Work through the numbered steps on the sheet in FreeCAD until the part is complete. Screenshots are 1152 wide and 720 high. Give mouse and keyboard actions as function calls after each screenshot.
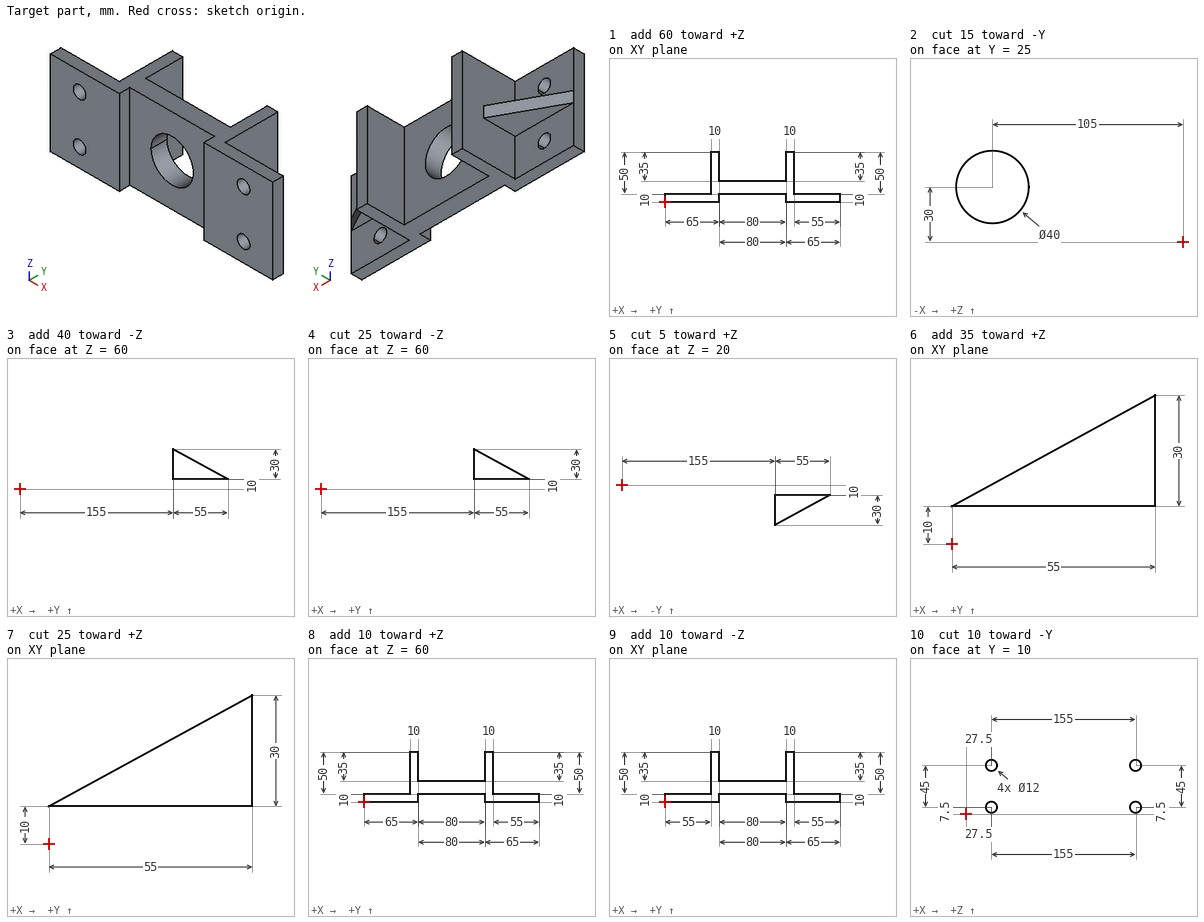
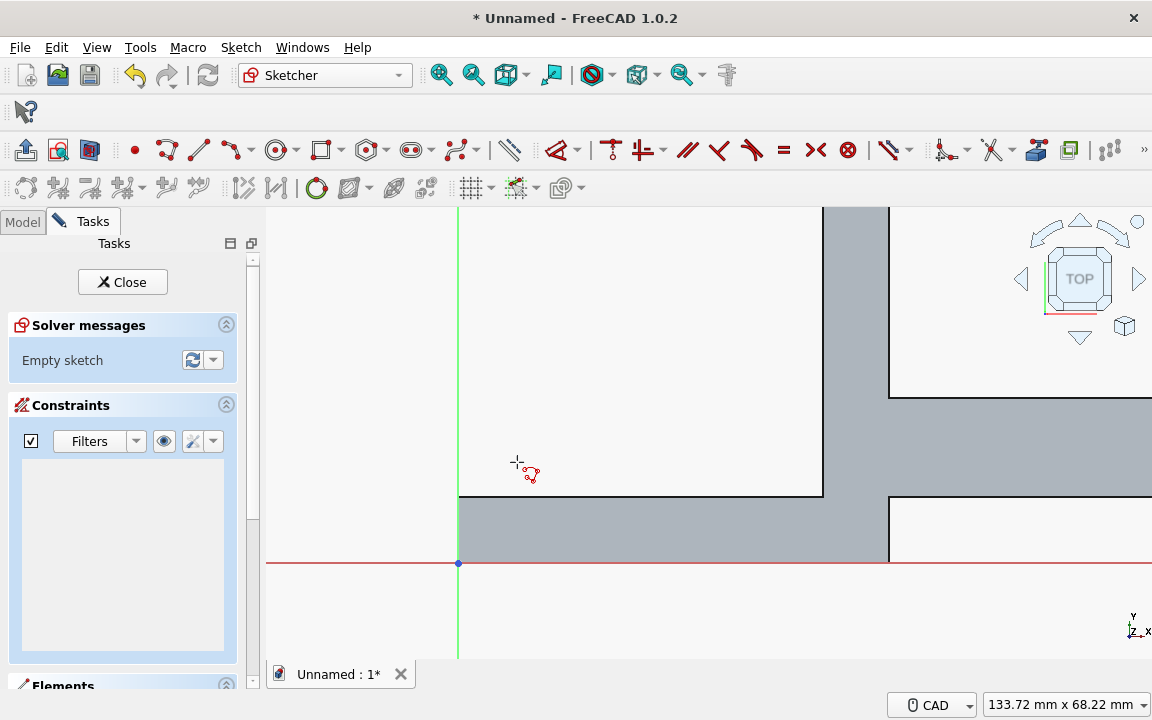
click(458, 497)
click(823, 298)
click(823, 497)
click(458, 498)
key(Escape)
key(Escape)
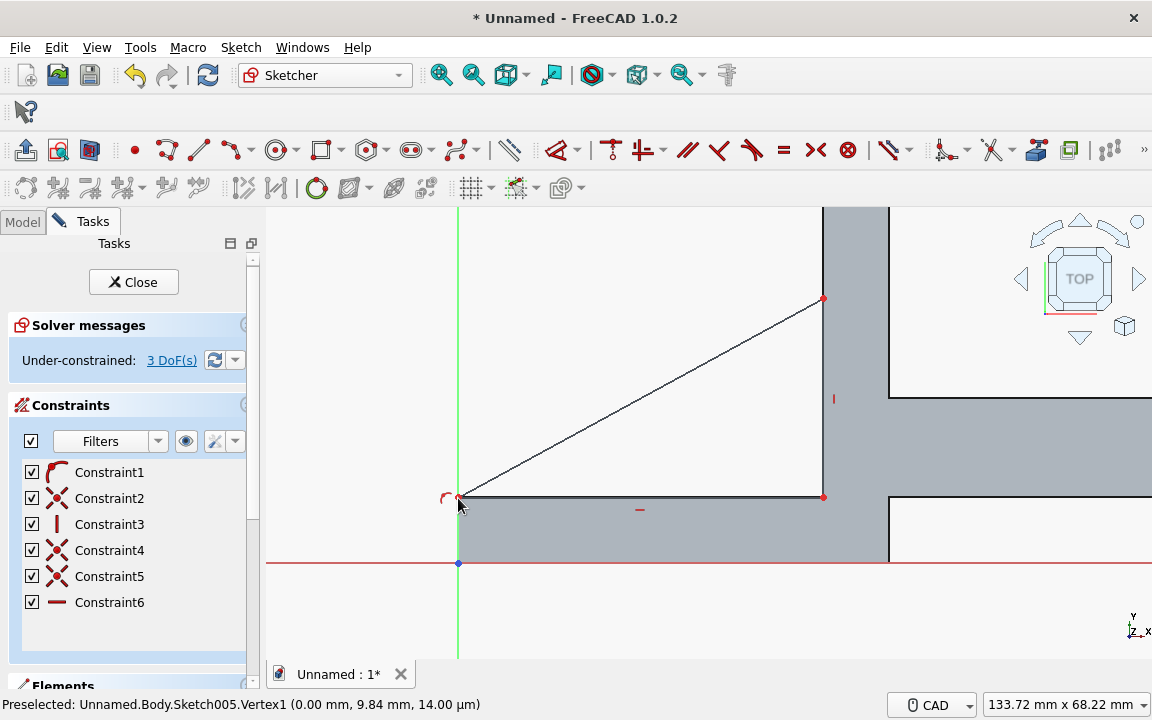
click(556, 150)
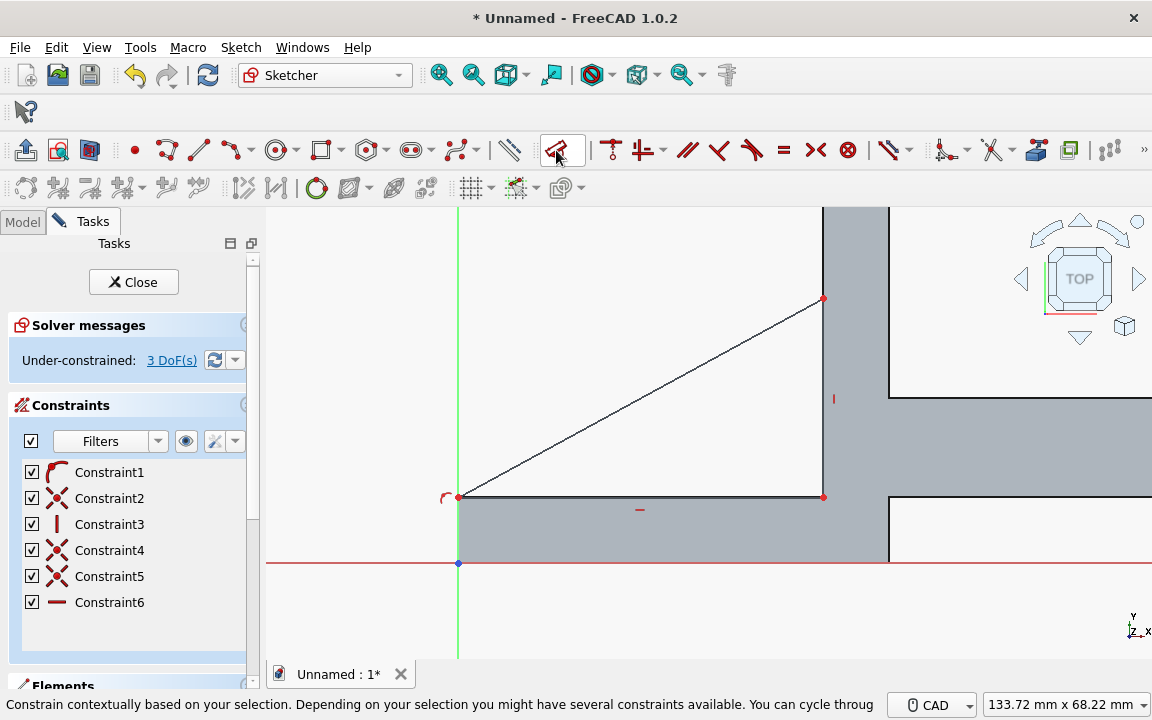
click(823, 359)
click(857, 399)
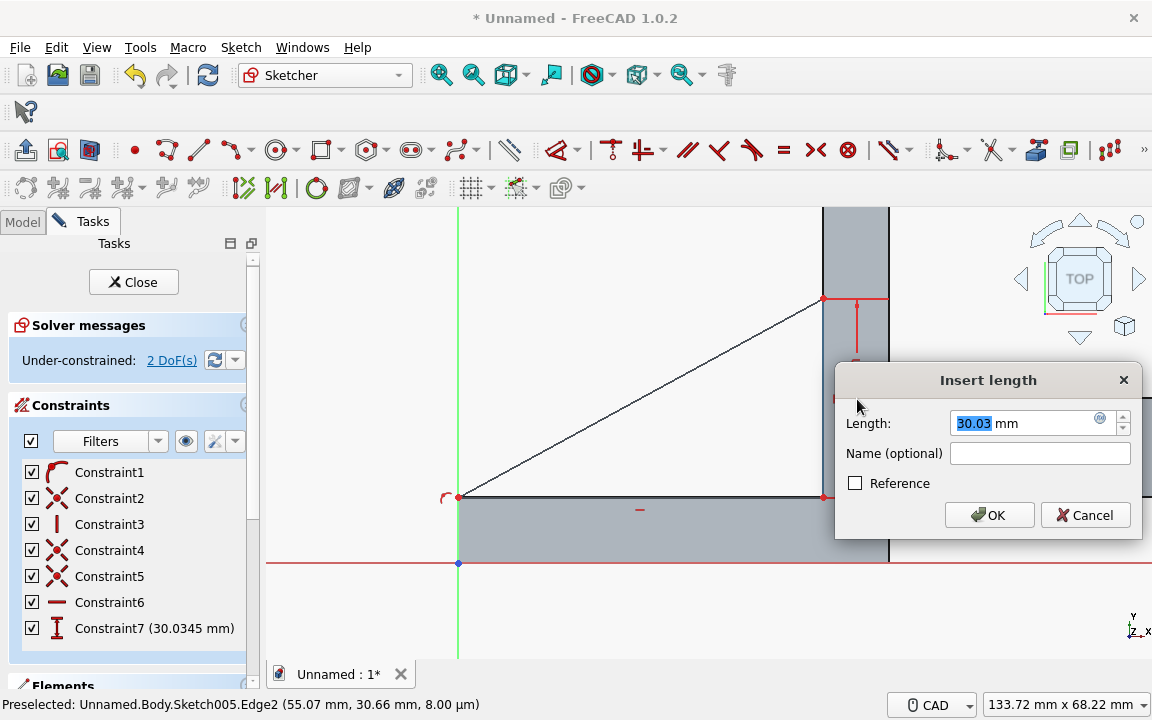
text(30)
key(Return)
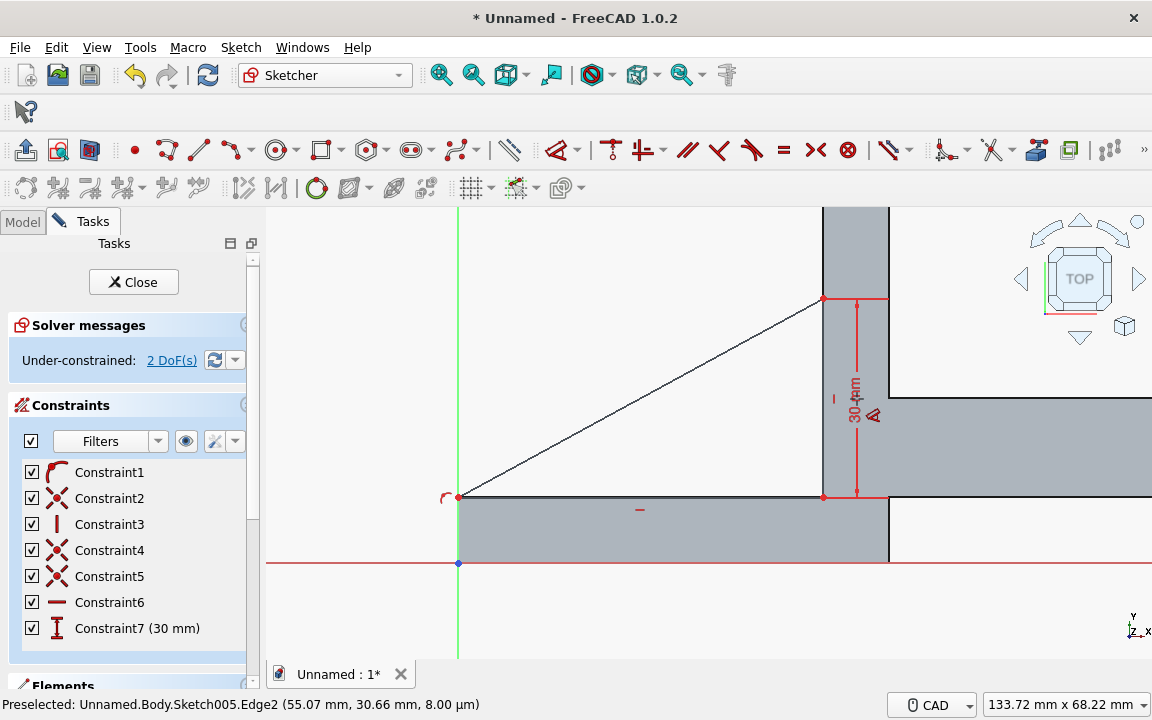
click(714, 498)
click(641, 532)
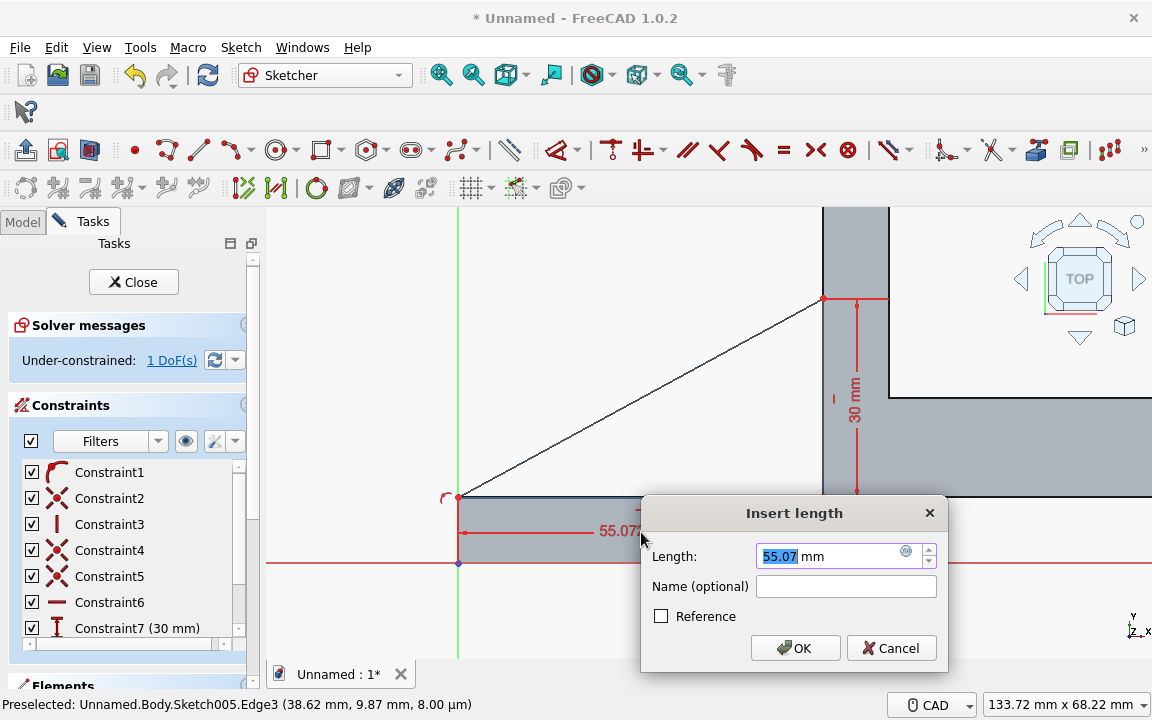
text(55)
key(Return)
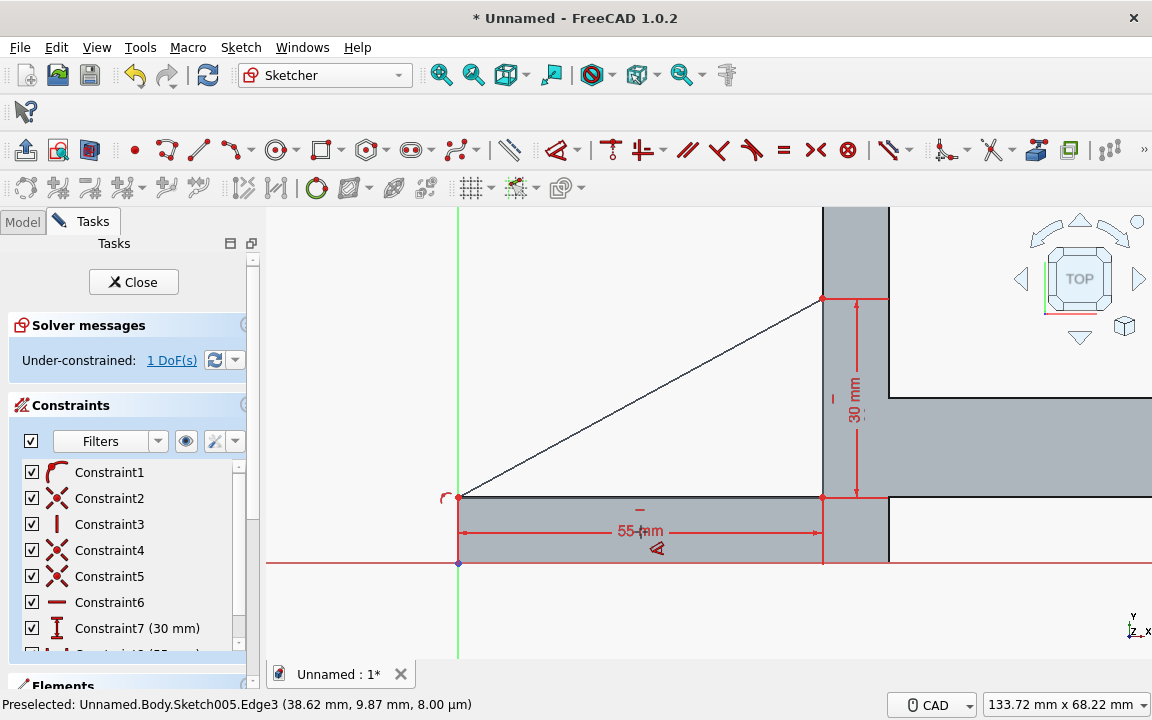
click(458, 498)
click(424, 530)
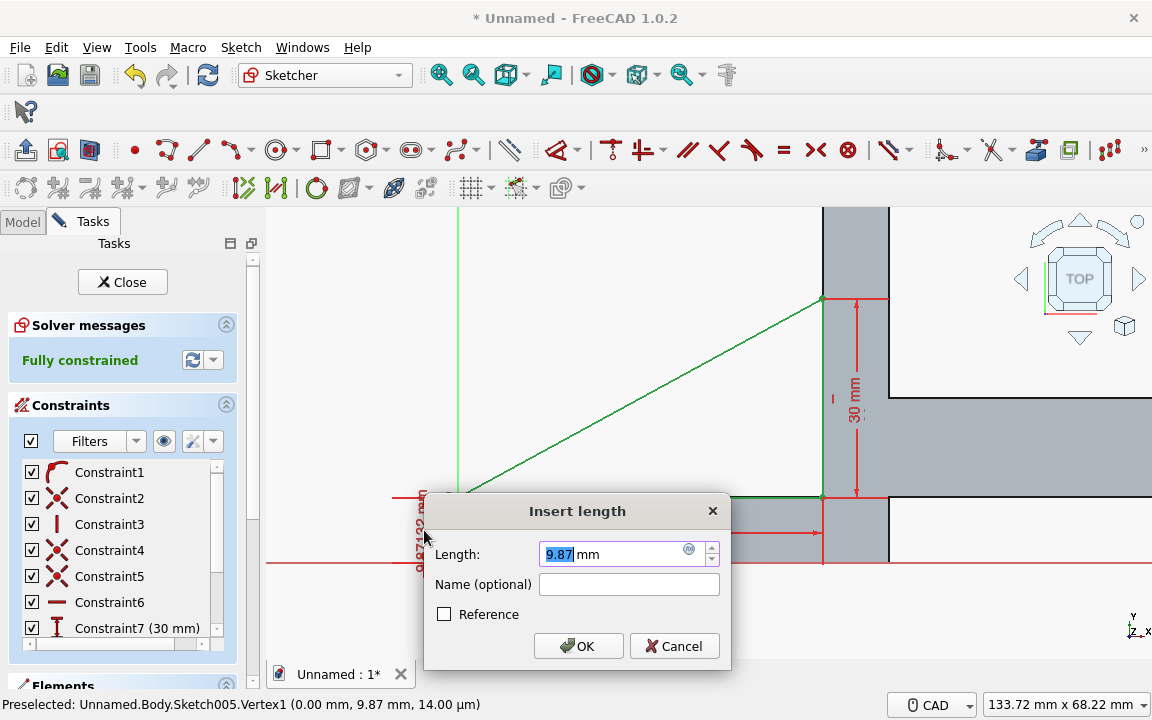
text(10)
key(Return)
key(Escape)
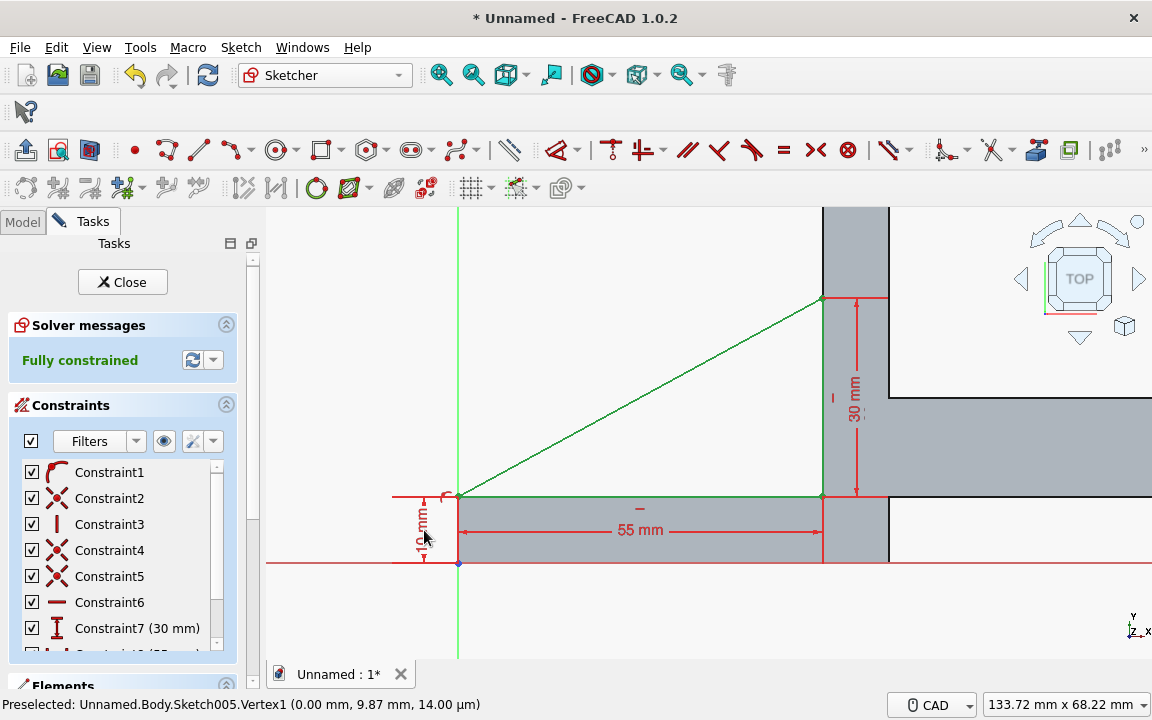
click(123, 282)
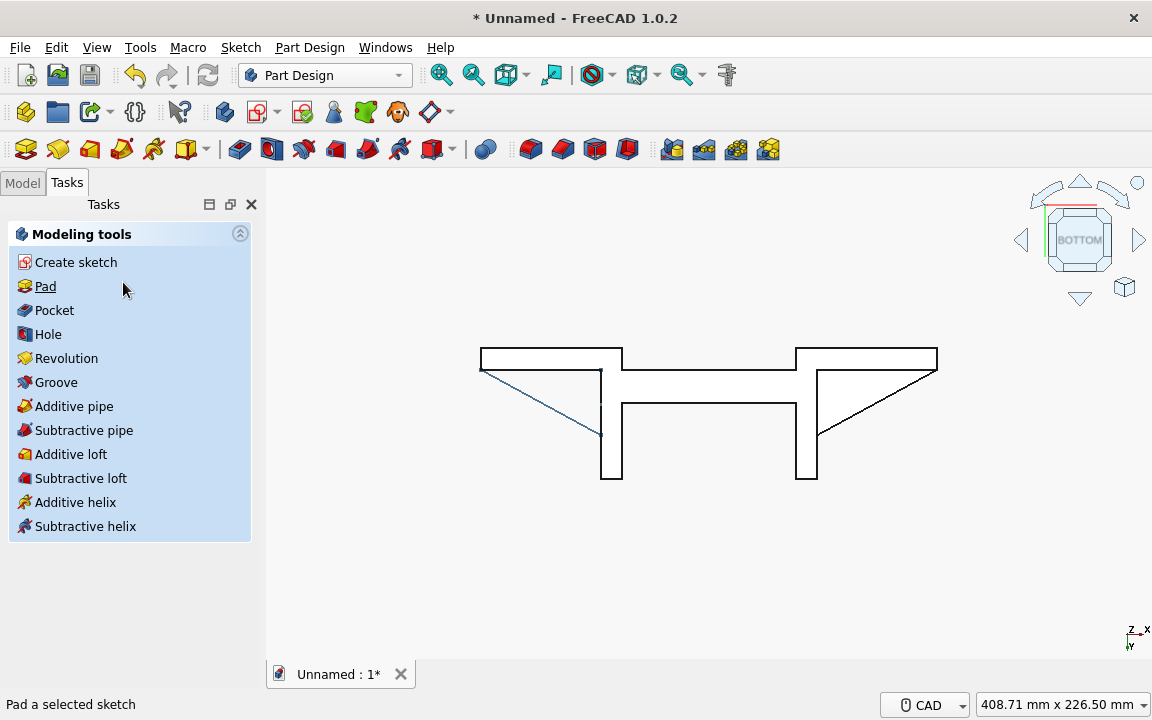
click(26, 150)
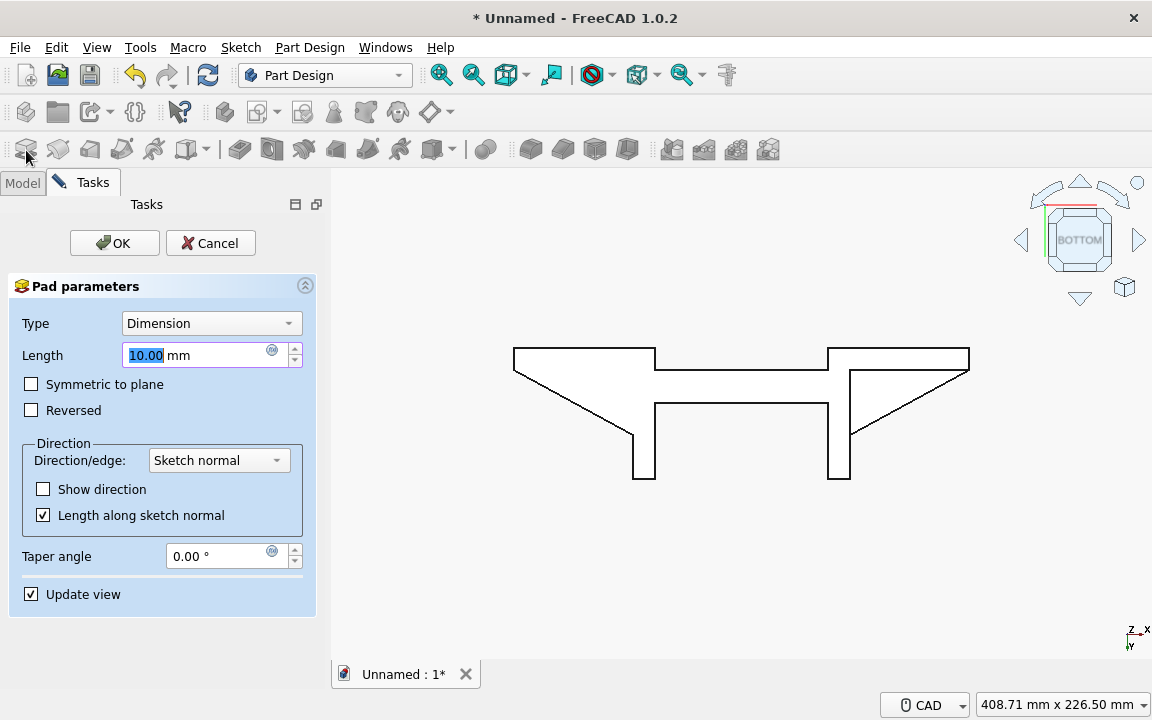
text(35)
key(Tab)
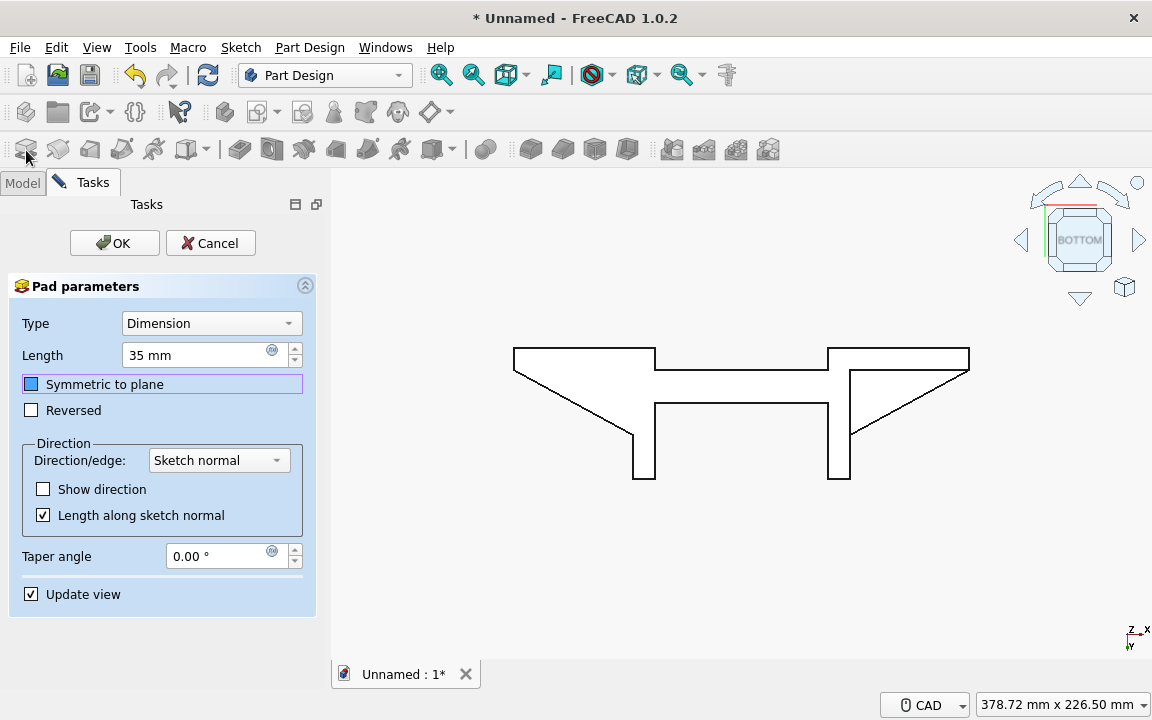
click(115, 243)